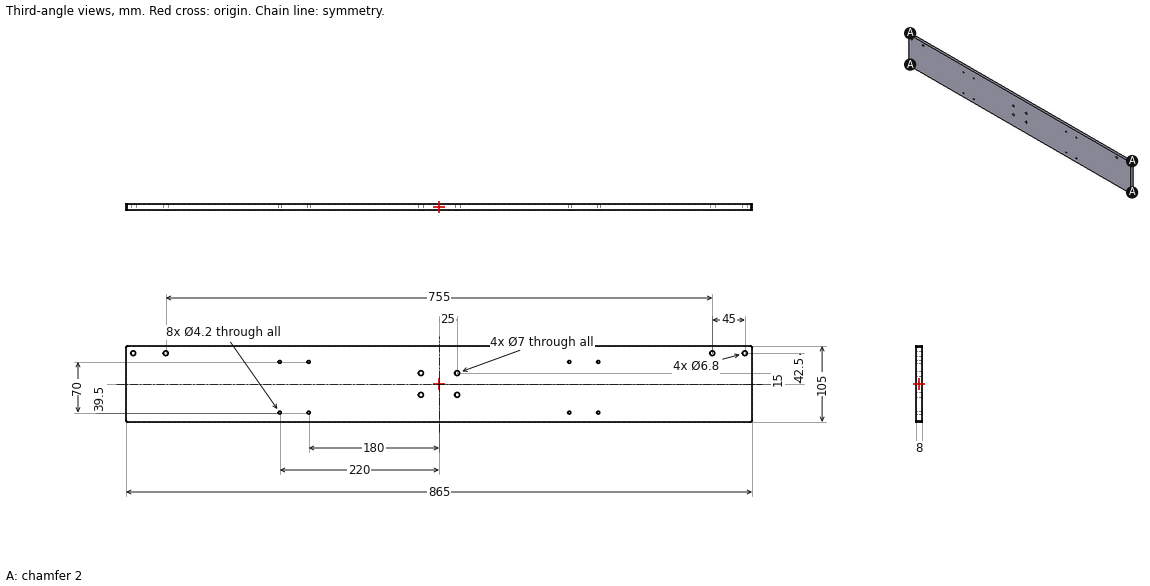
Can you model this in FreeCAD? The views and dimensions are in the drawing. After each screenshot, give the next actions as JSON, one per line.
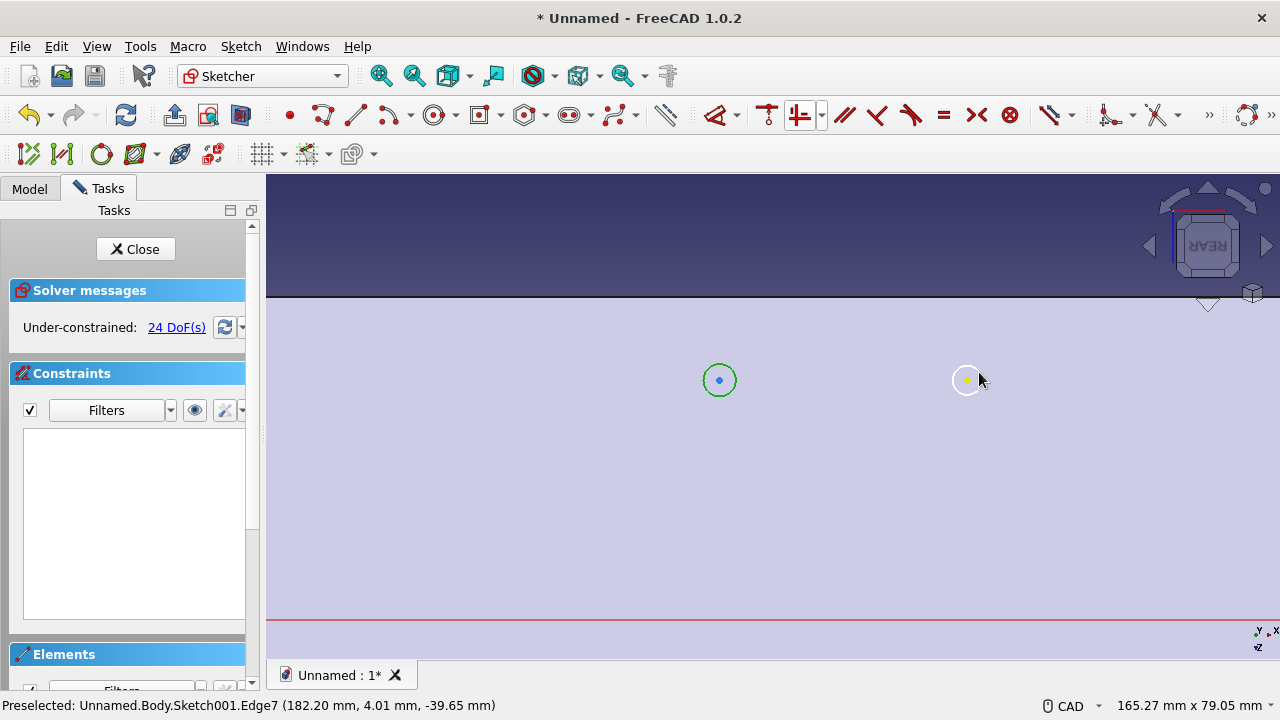
{"action": "left_click", "coordinate": [978, 370]}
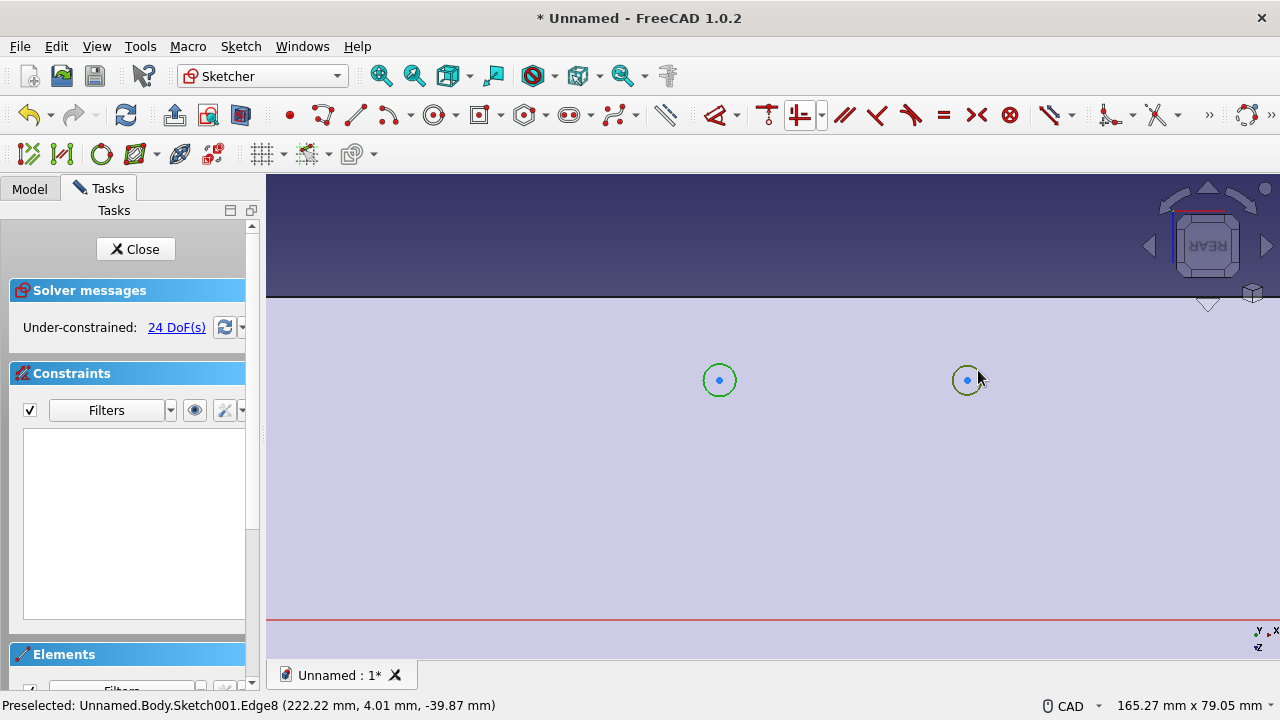
{"action": "key", "text": "e"}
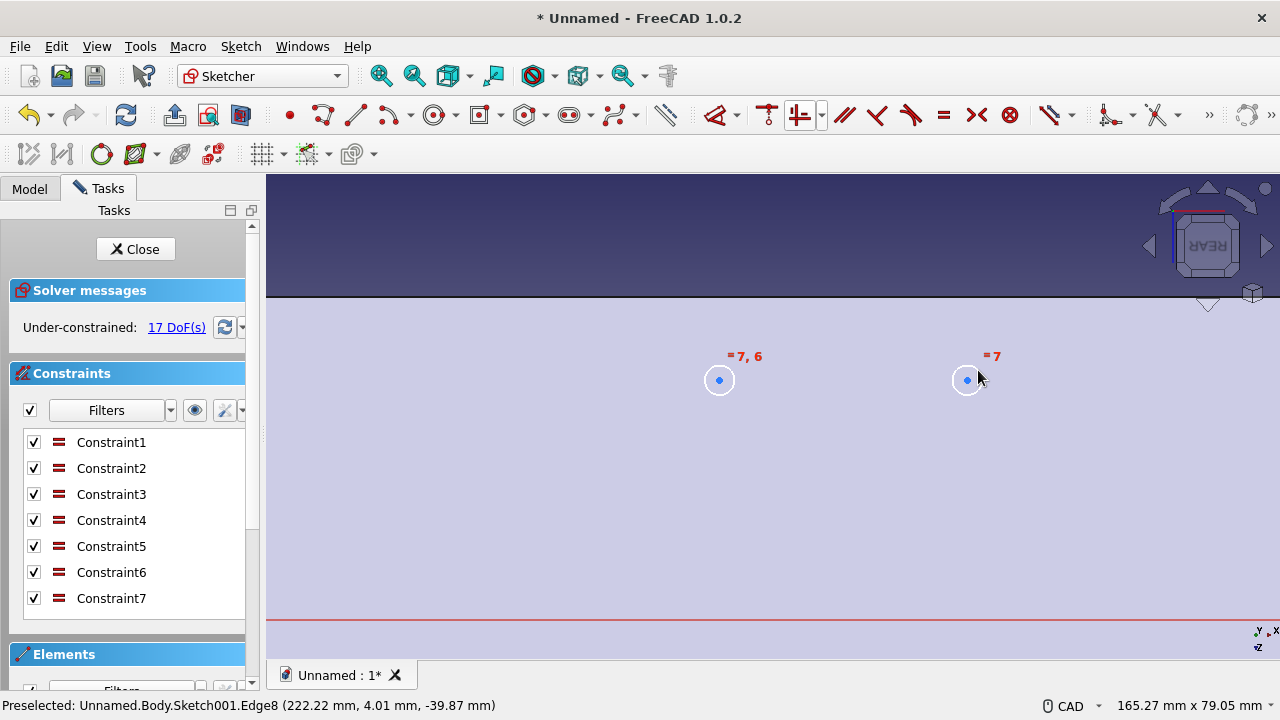
{"action": "scroll", "coordinate": [979, 372], "scroll_direction": "down", "scroll_amount": 8}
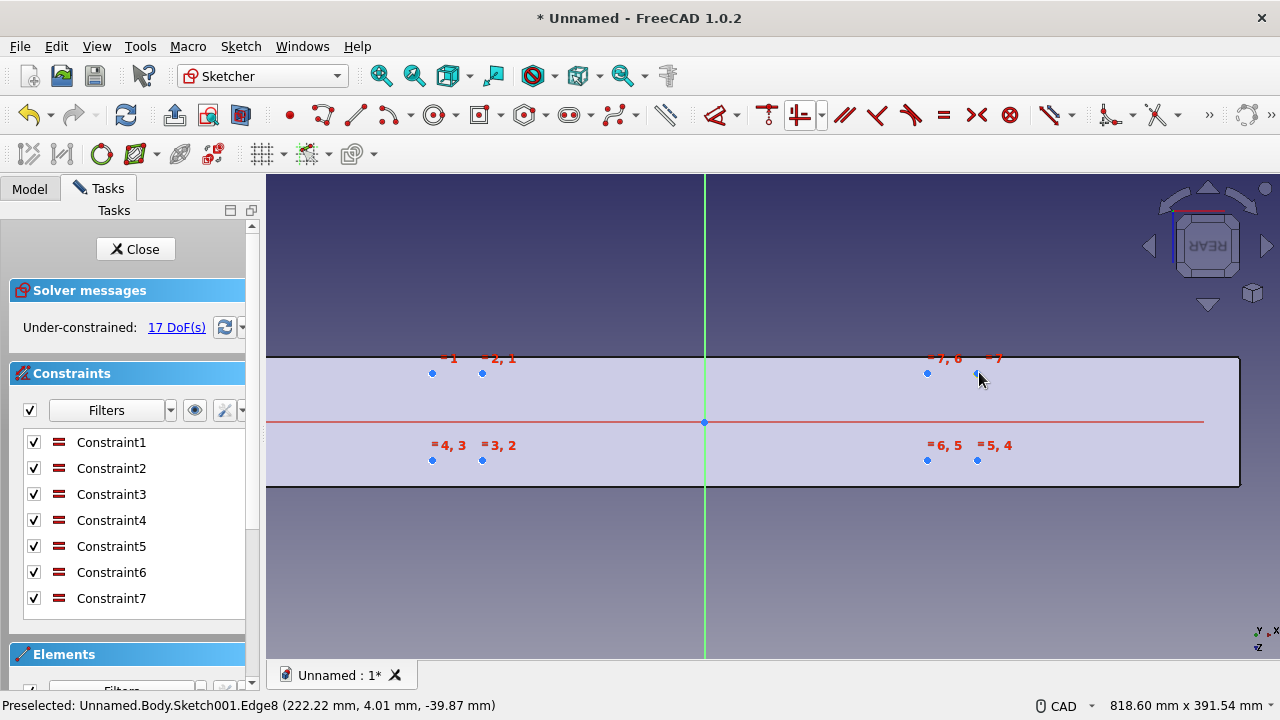
{"action": "left_click", "coordinate": [432, 461]}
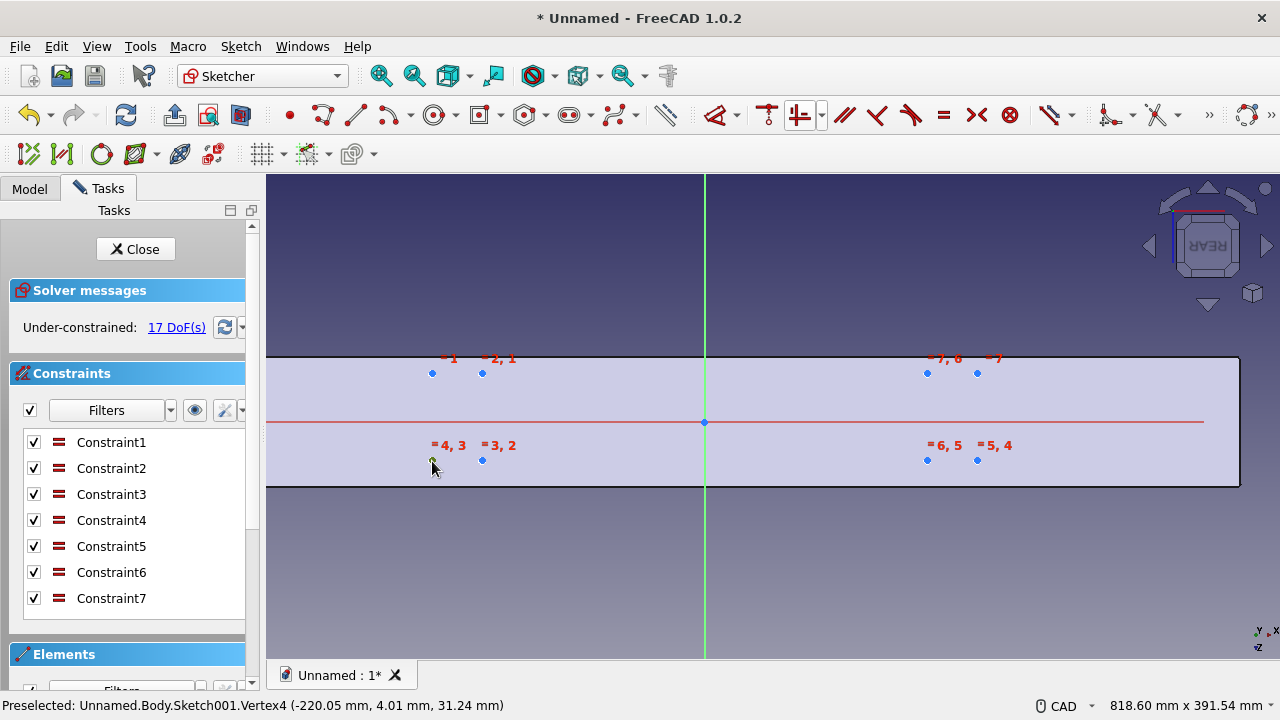
{"action": "left_click", "coordinate": [977, 461]}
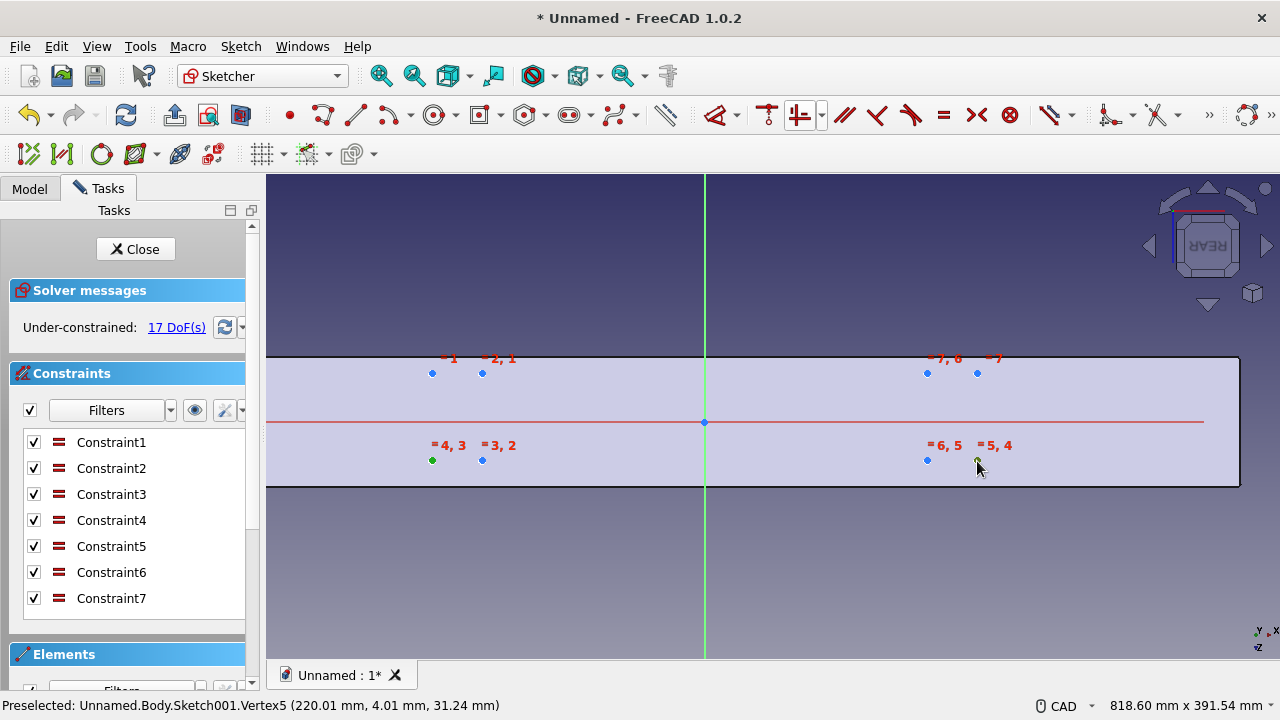
{"action": "left_click", "coordinate": [705, 600]}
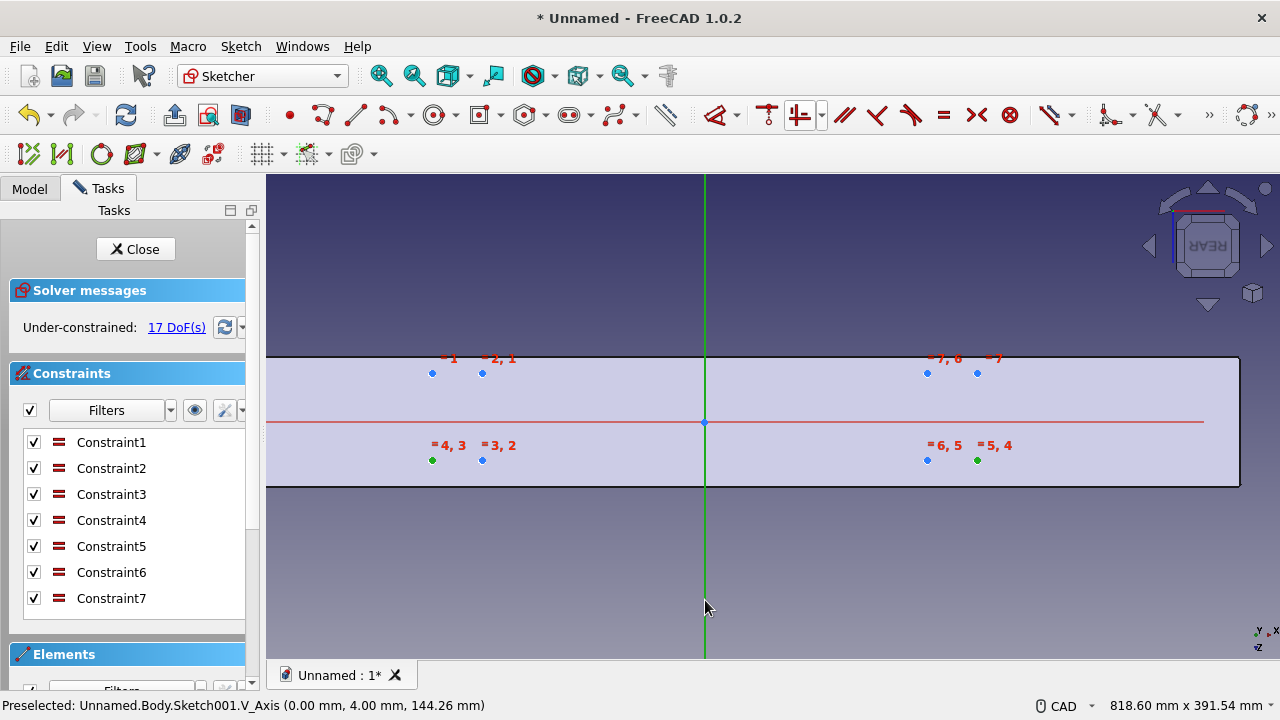
{"action": "left_click", "coordinate": [977, 116]}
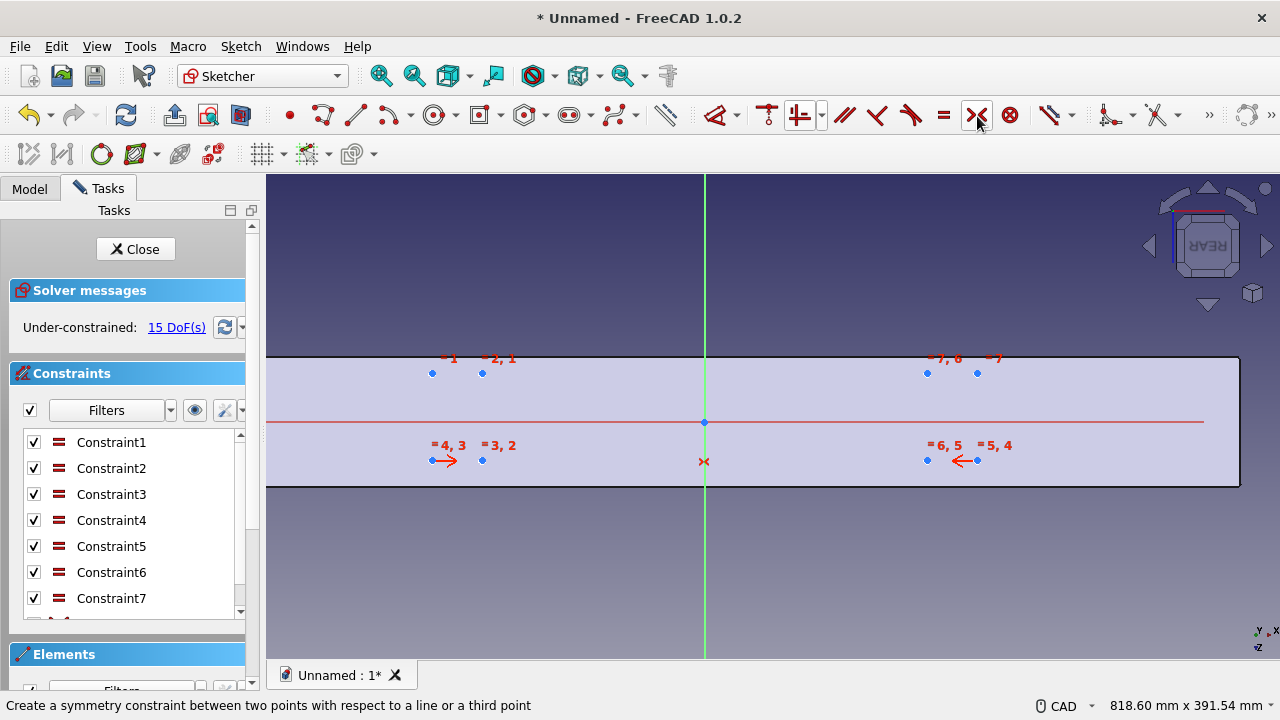
{"action": "left_click", "coordinate": [482, 461]}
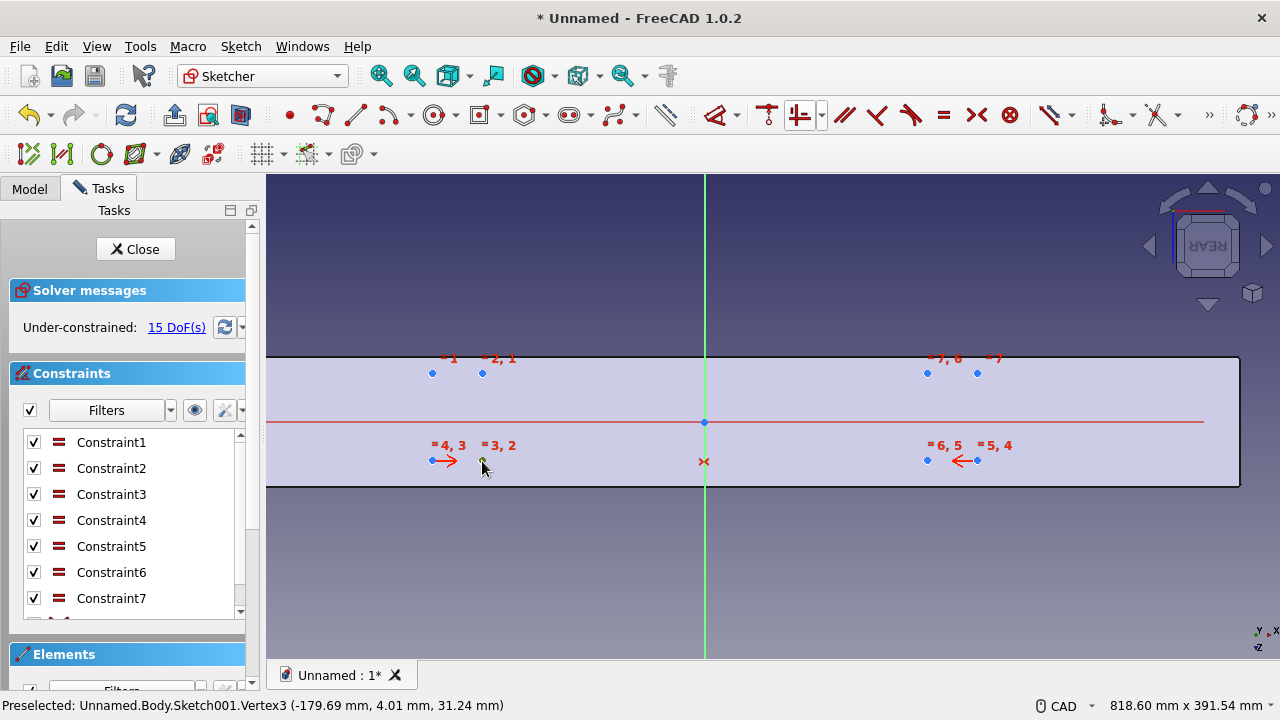
{"action": "left_click", "coordinate": [927, 461]}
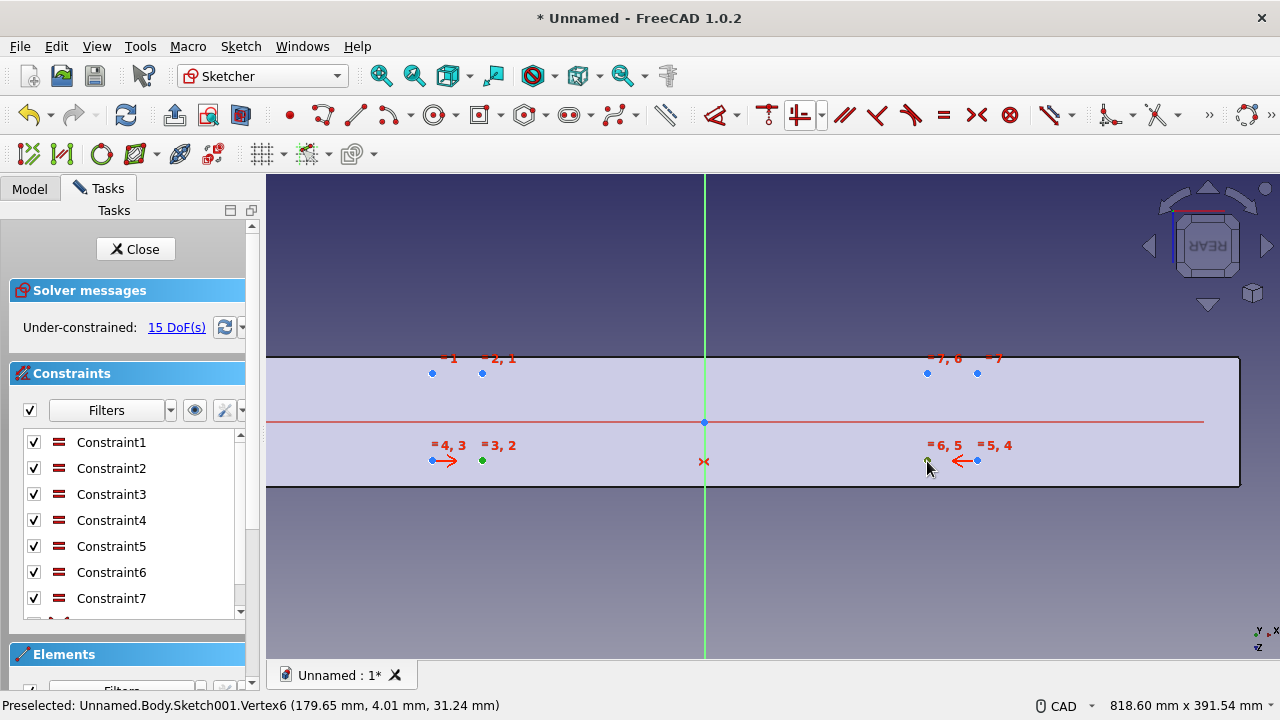
{"action": "left_click", "coordinate": [705, 600]}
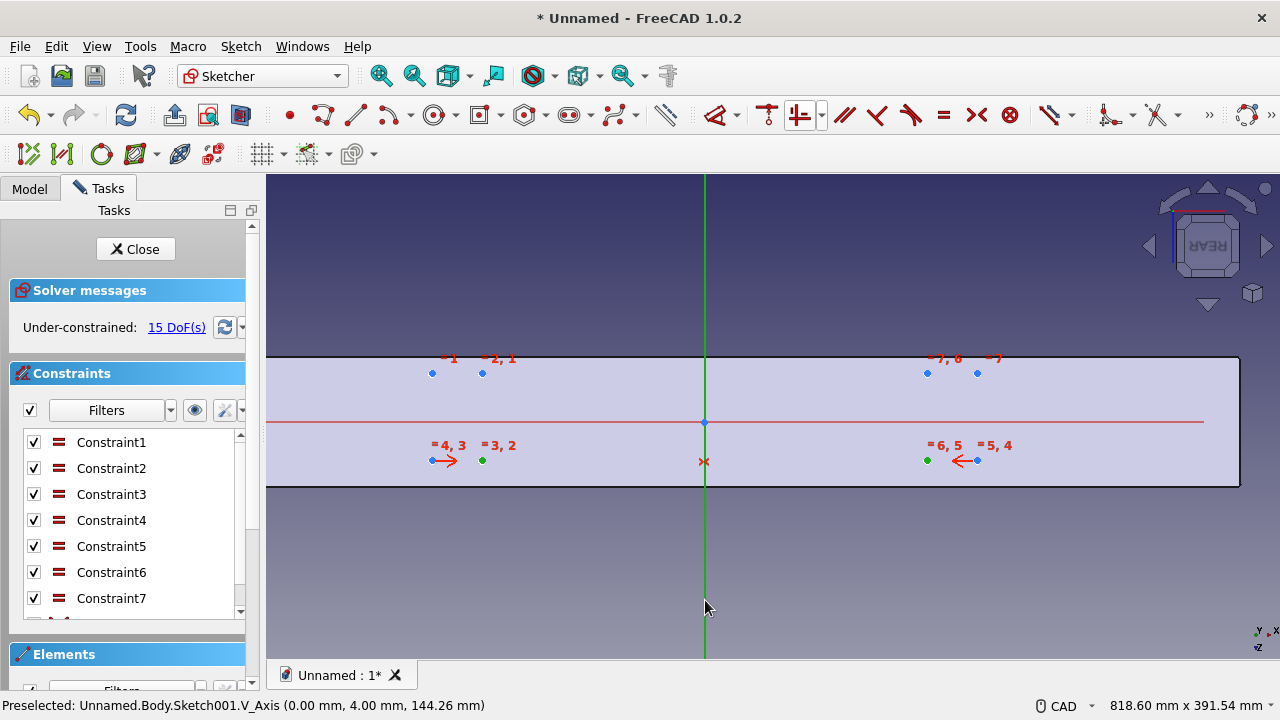
{"action": "key", "text": "s"}